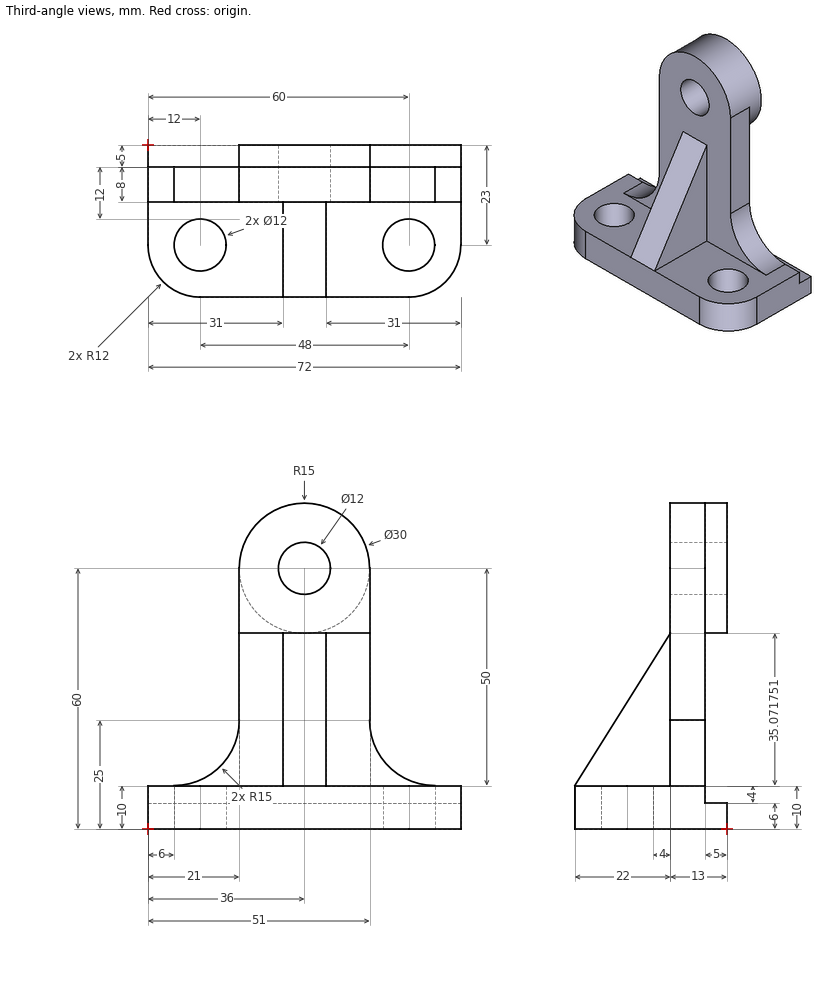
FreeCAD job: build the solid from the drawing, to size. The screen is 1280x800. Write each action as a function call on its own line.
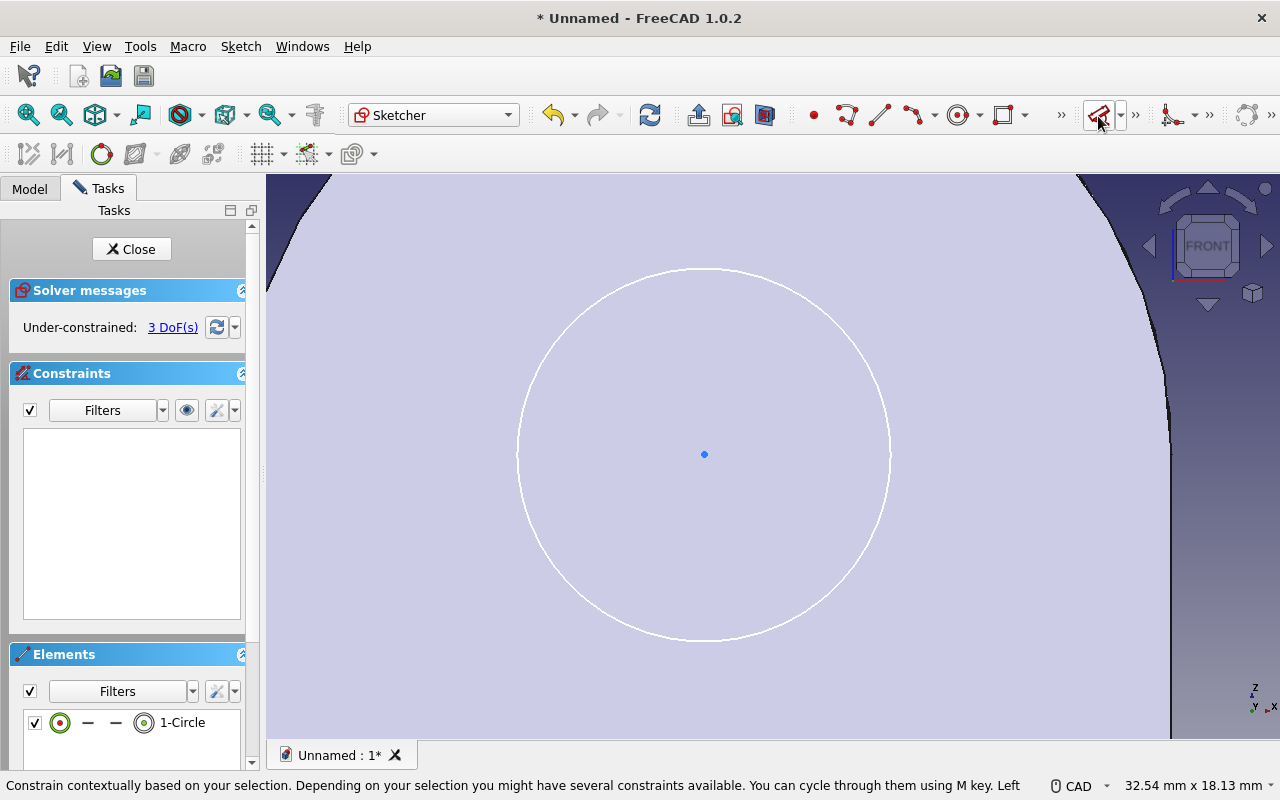
click(836, 323)
click(859, 300)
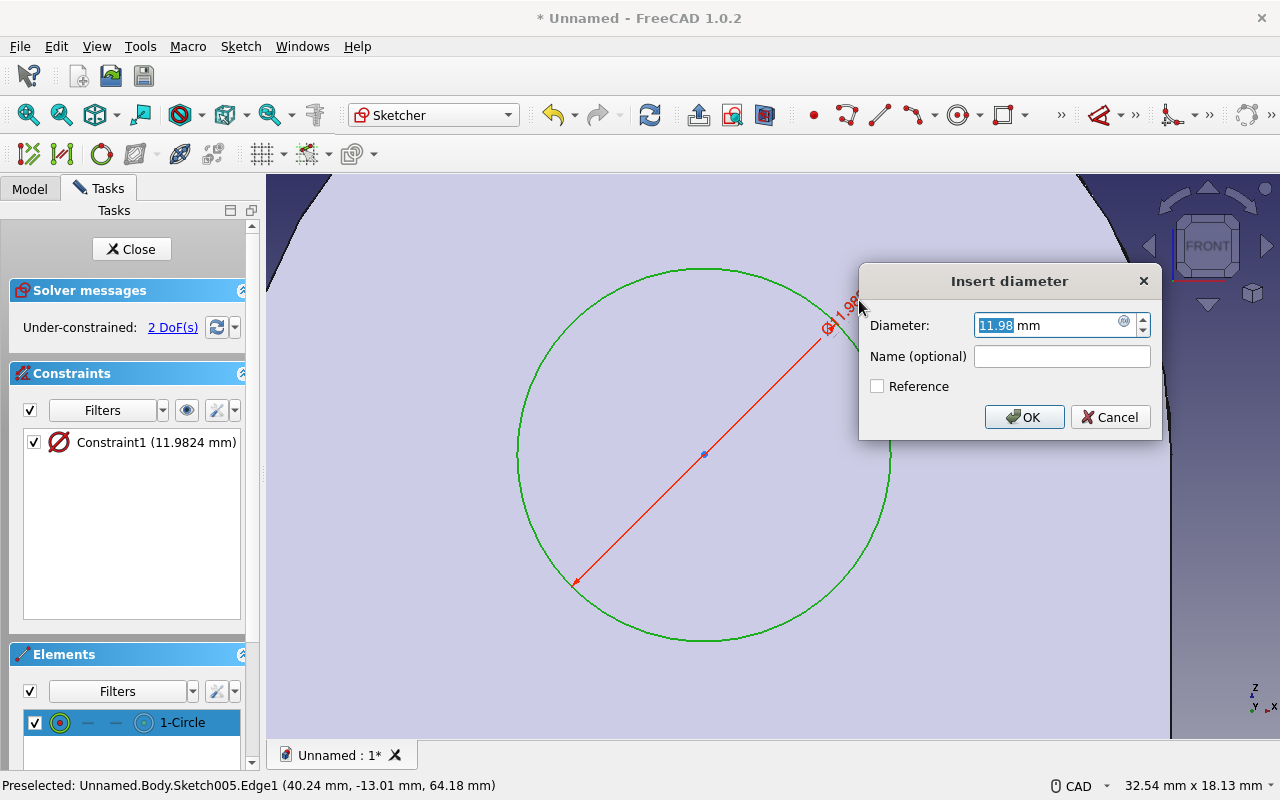
text(12)
key(Return)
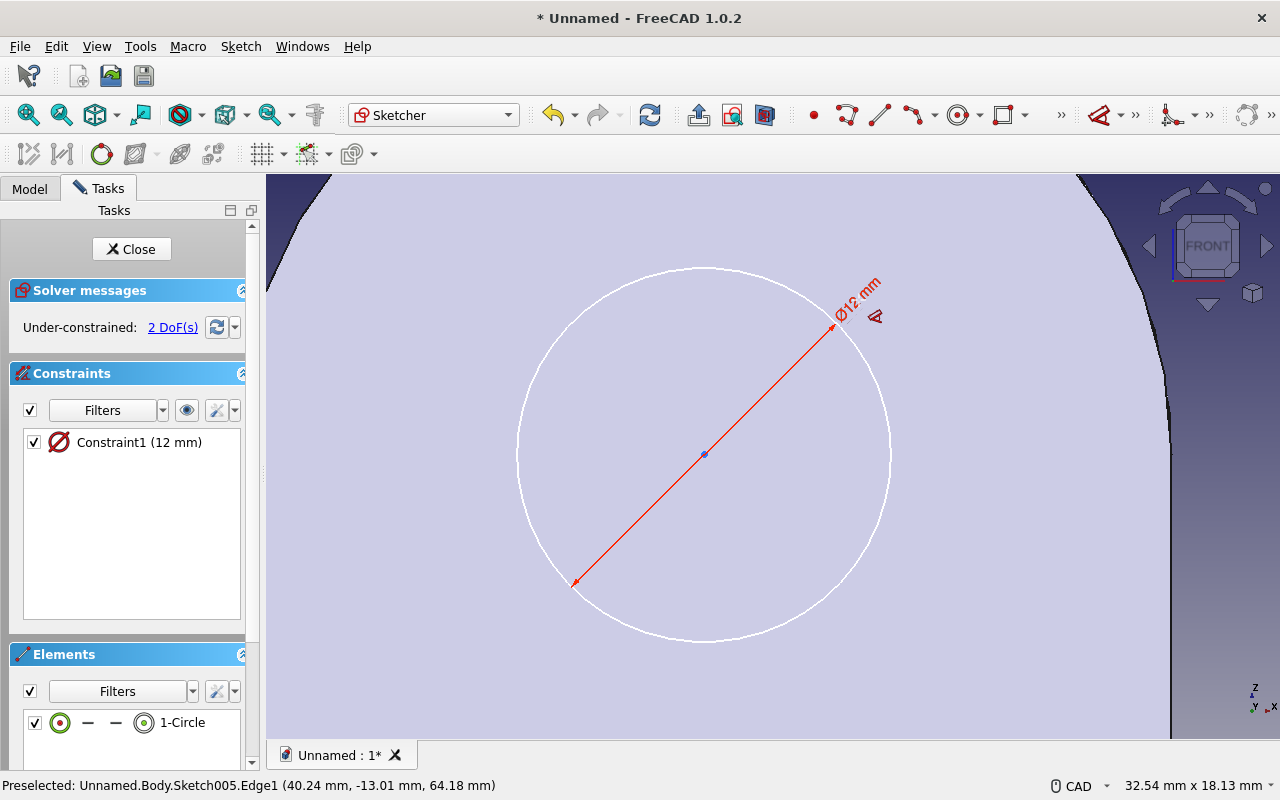
click(704, 455)
click(499, 421)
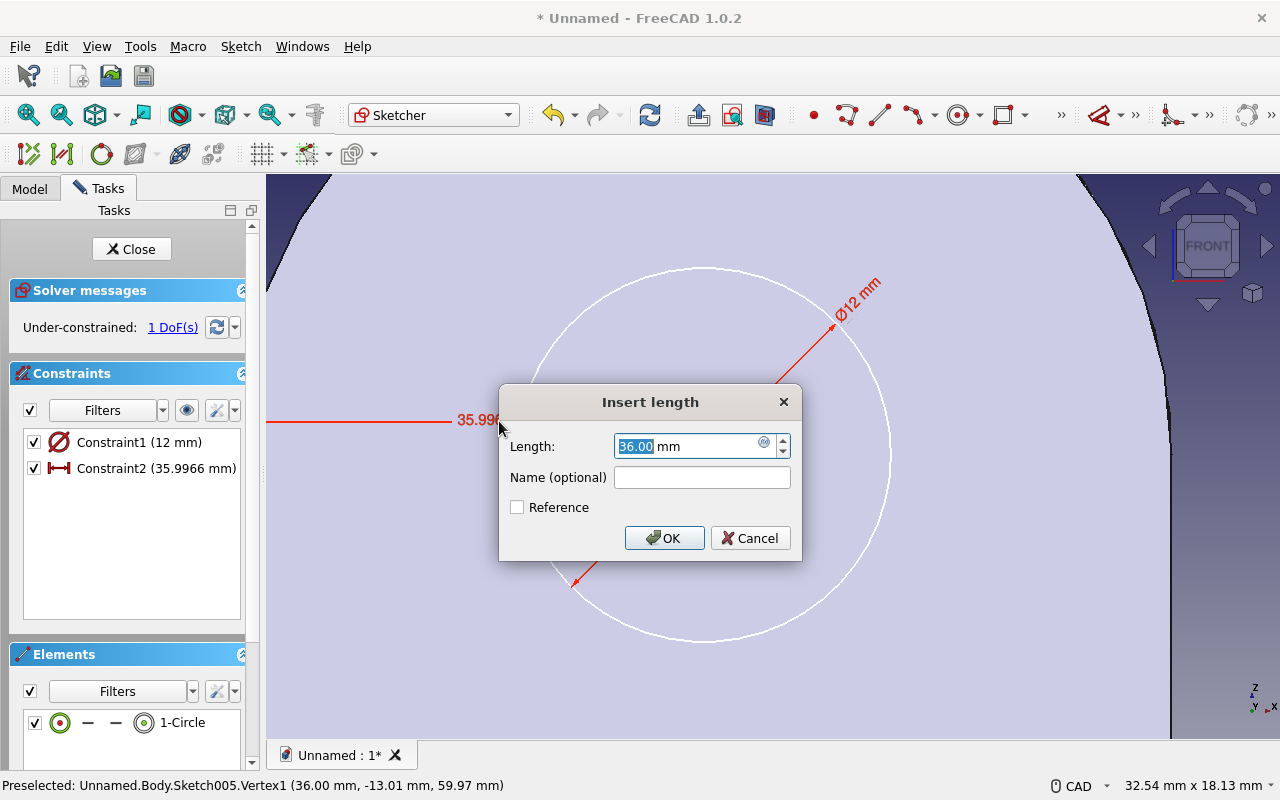
text(36)
key(Return)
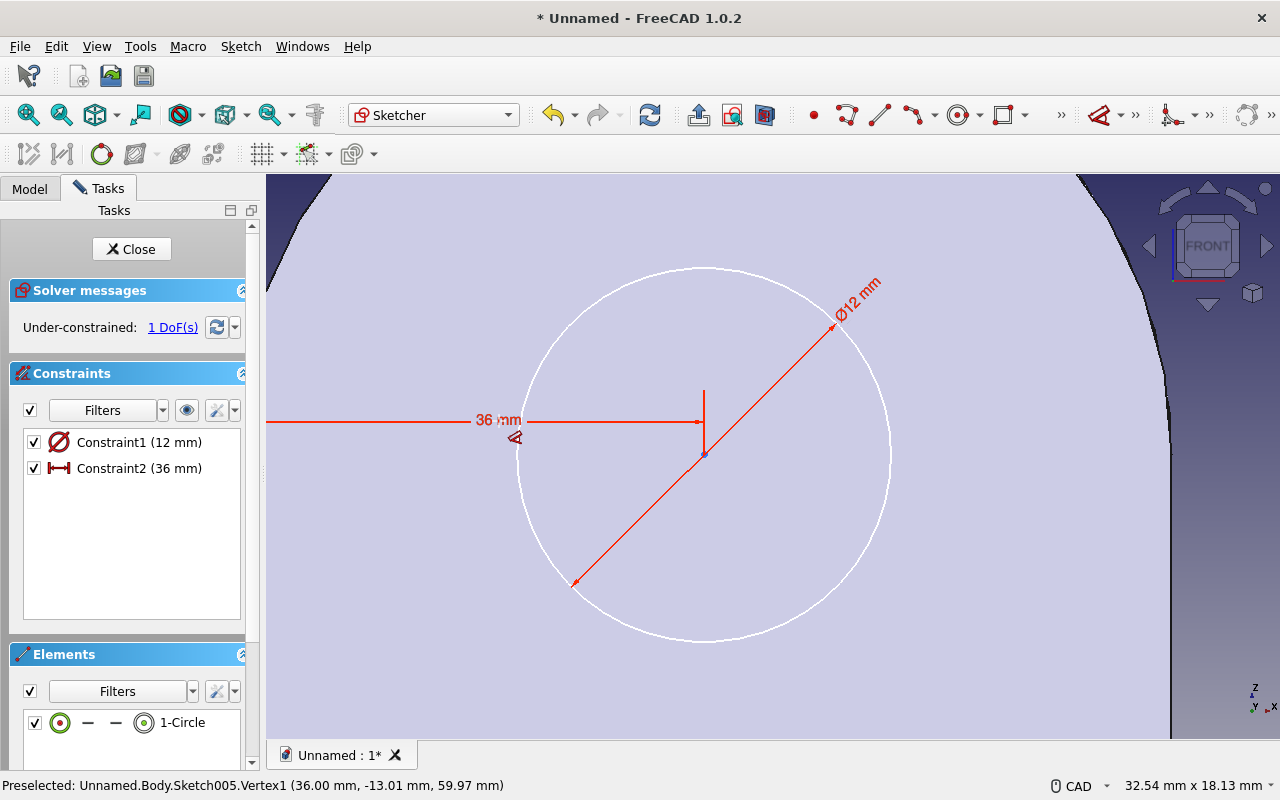
click(704, 455)
click(738, 583)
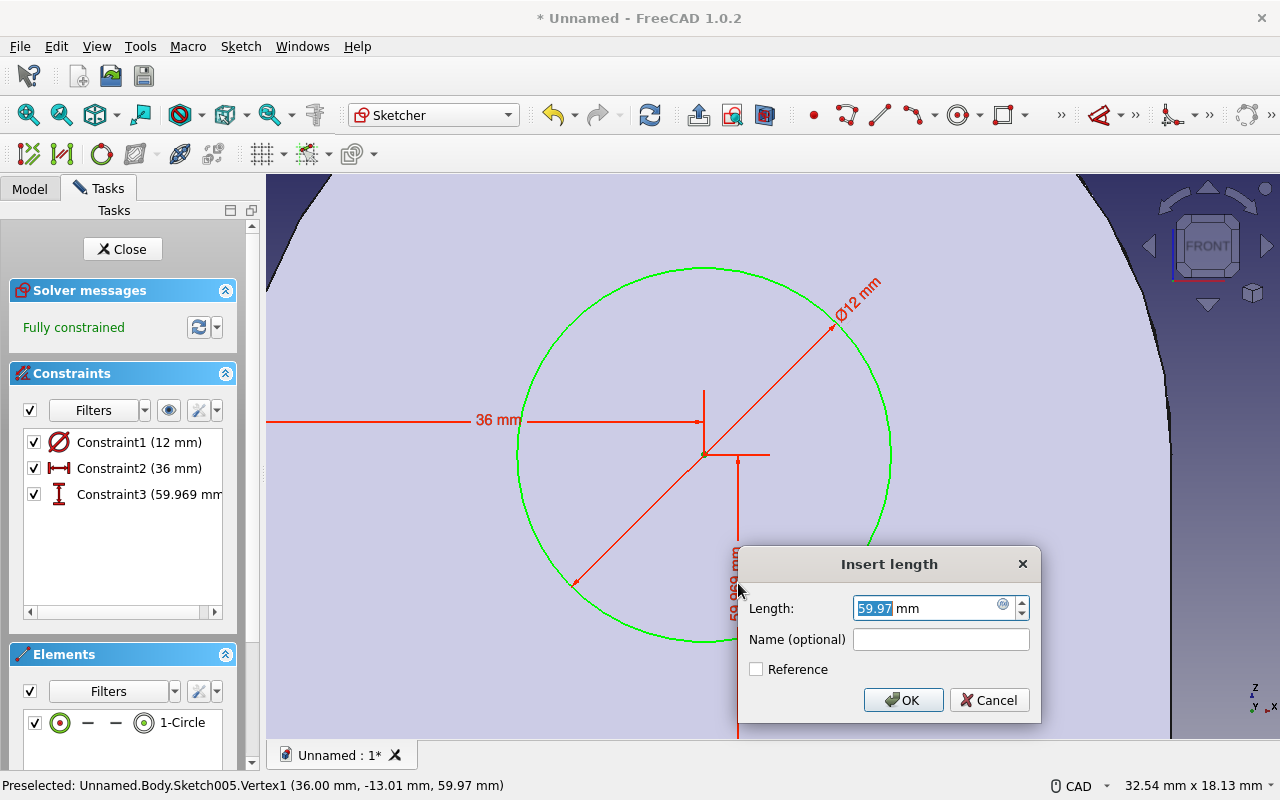
text(60)
key(Return)
key(Escape)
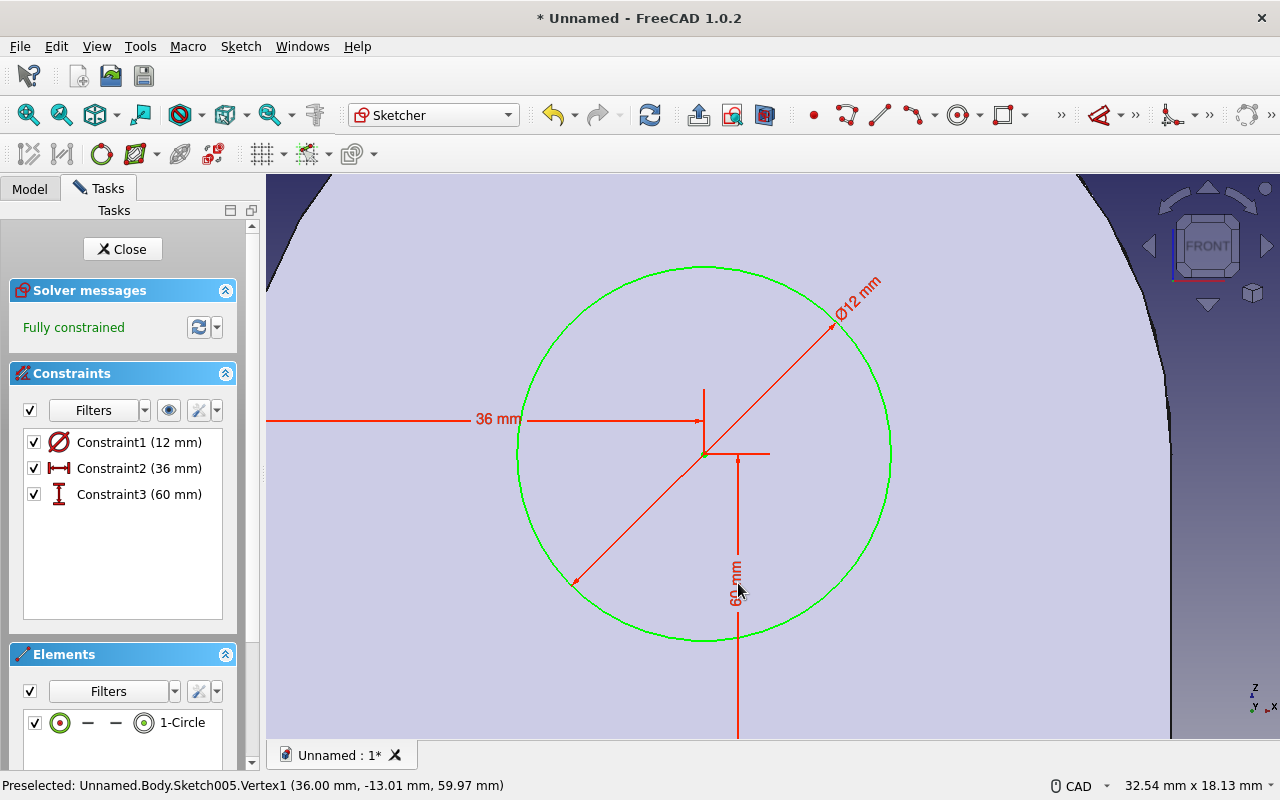
click(123, 249)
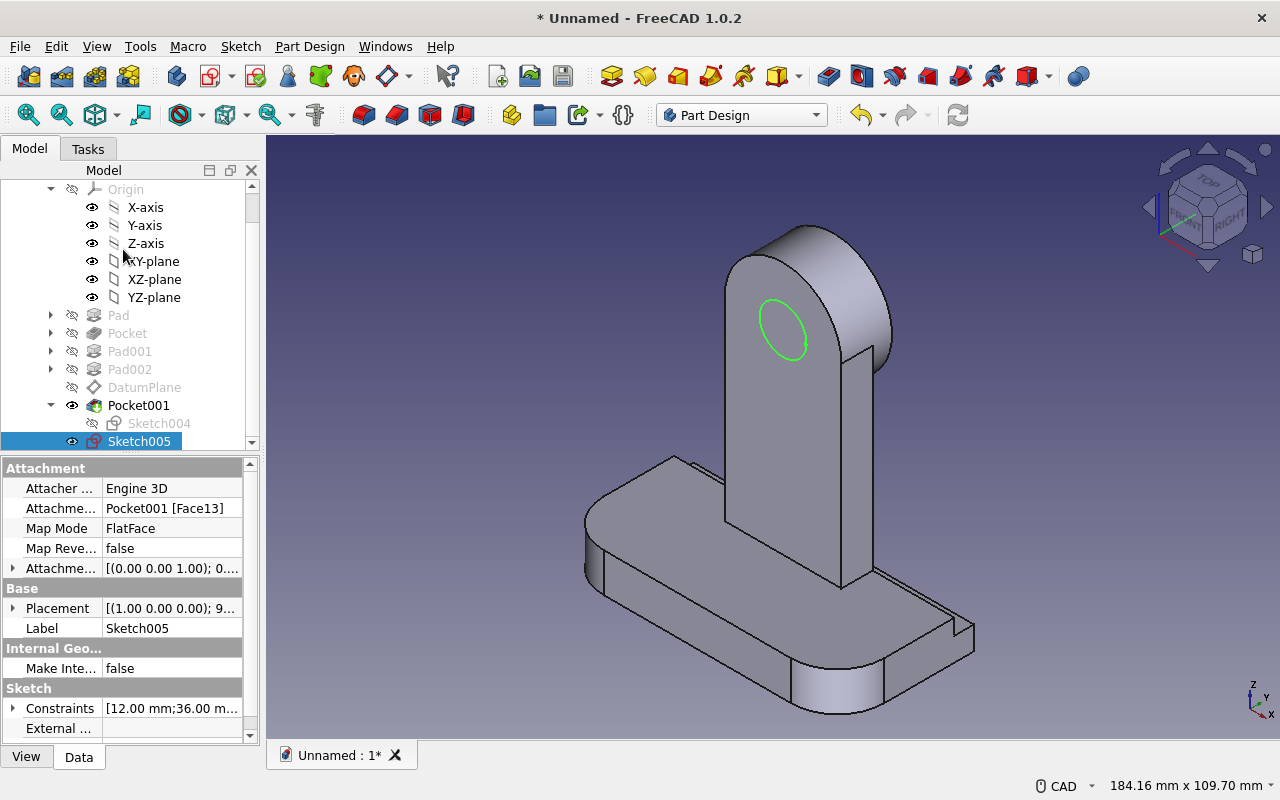
click(829, 76)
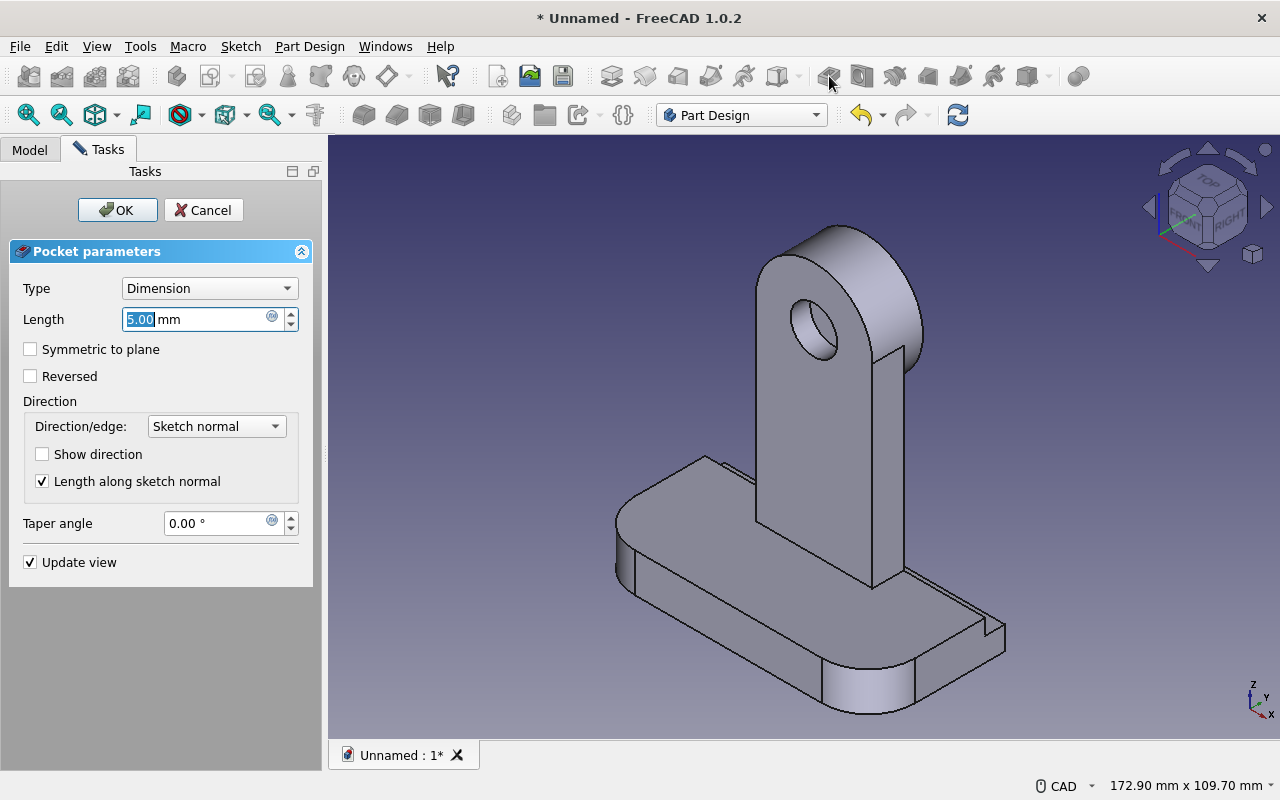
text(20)
key(Tab)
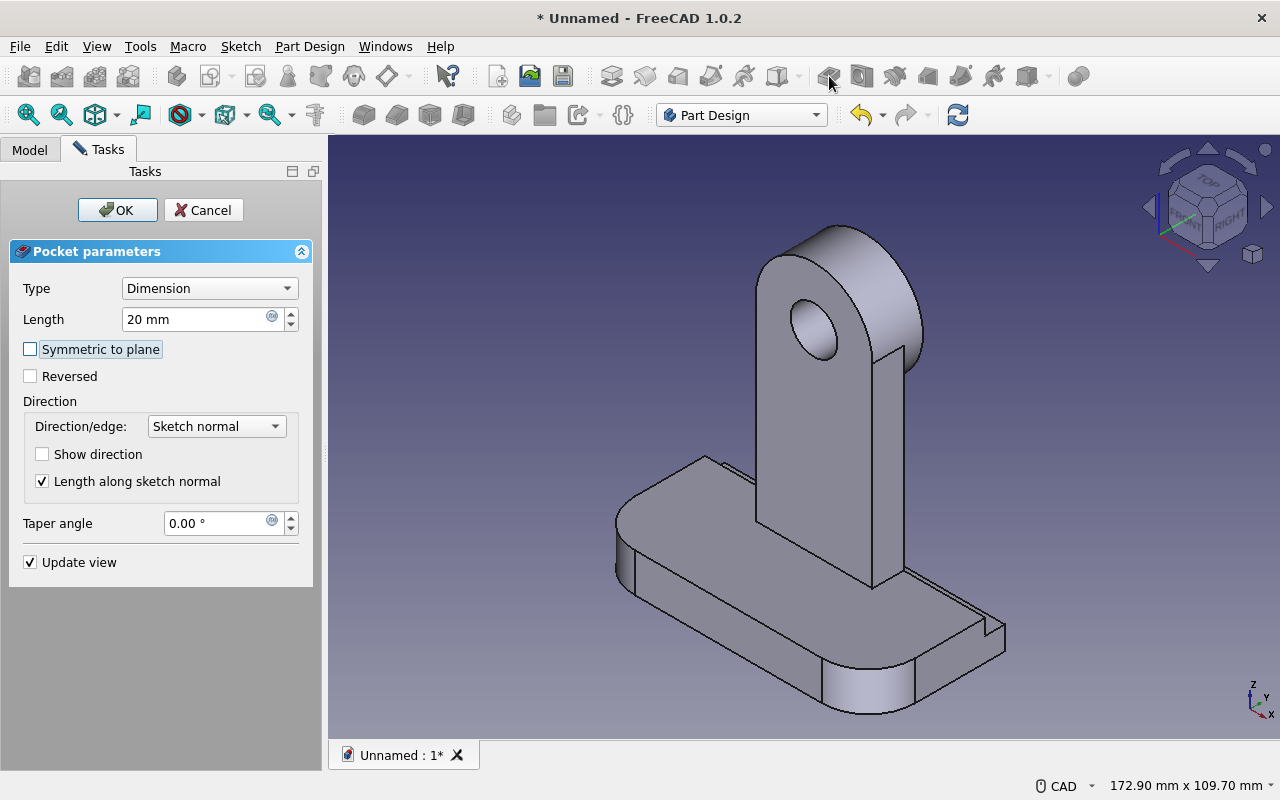
click(118, 210)